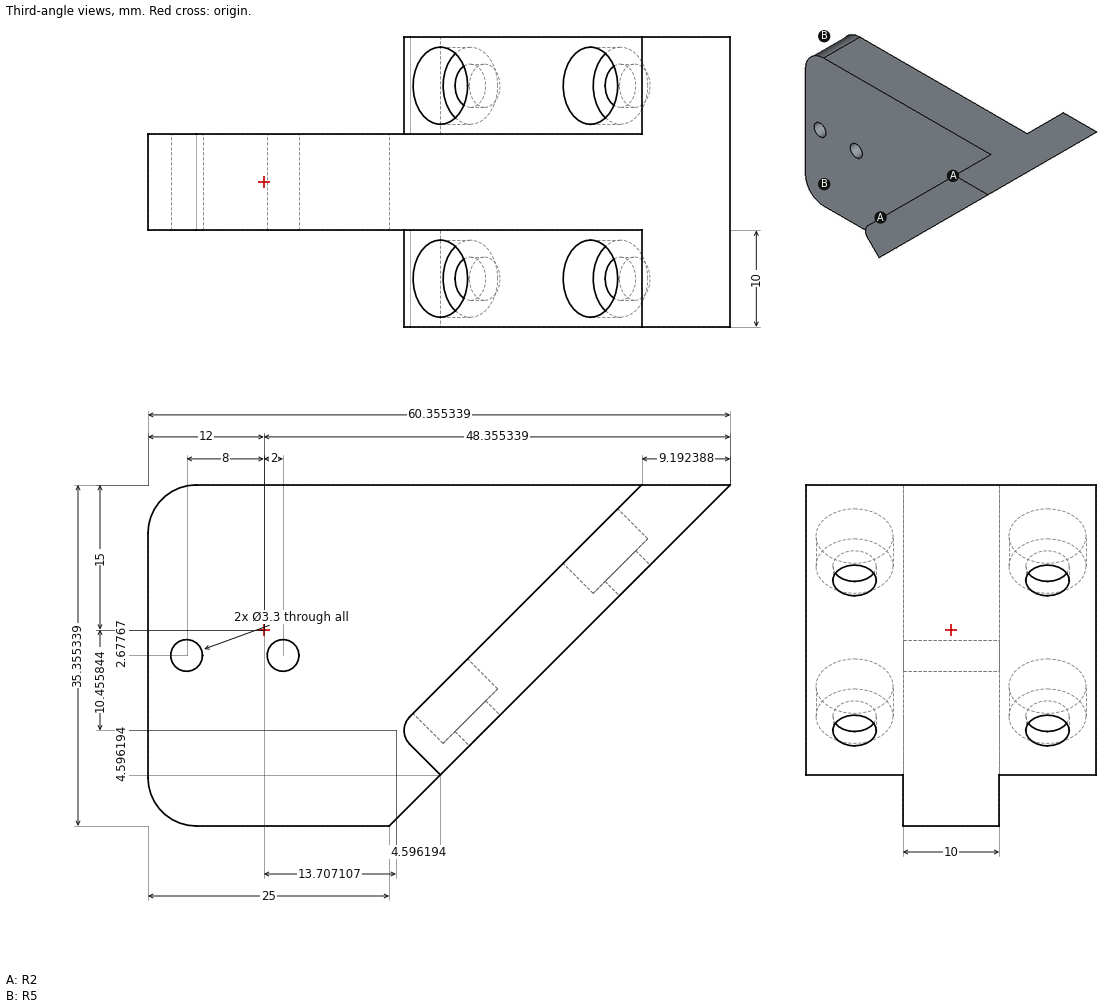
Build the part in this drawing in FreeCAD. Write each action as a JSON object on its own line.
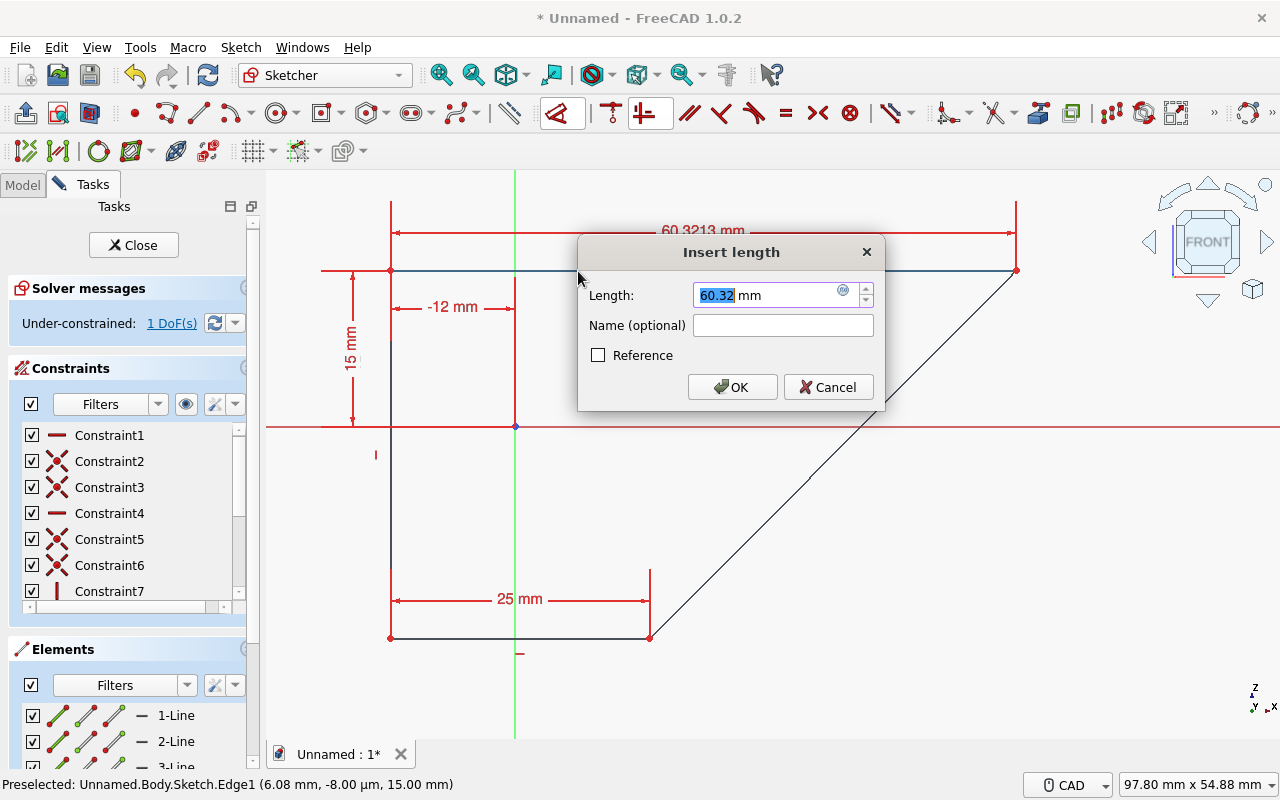
{"action": "type", "text": "60.355339"}
{"action": "key", "text": "Return"}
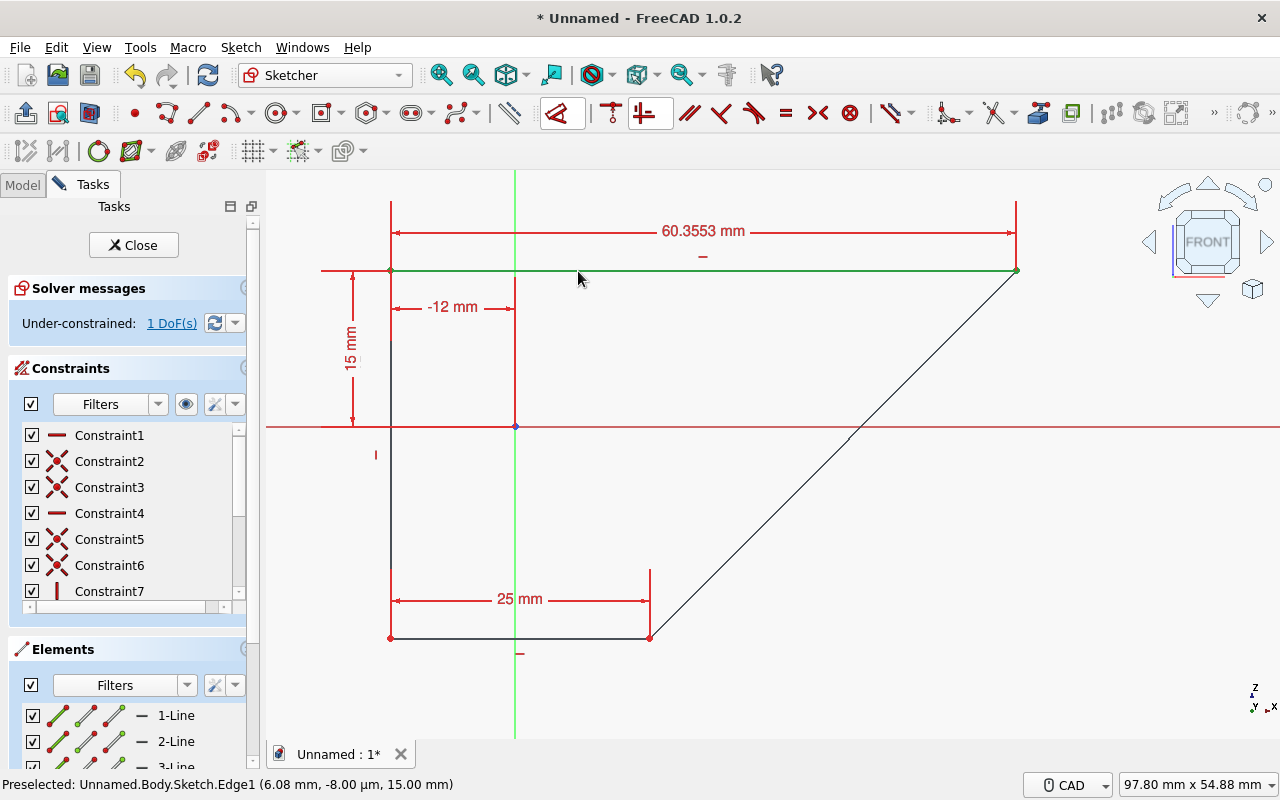
{"action": "left_click", "coordinate": [391, 529]}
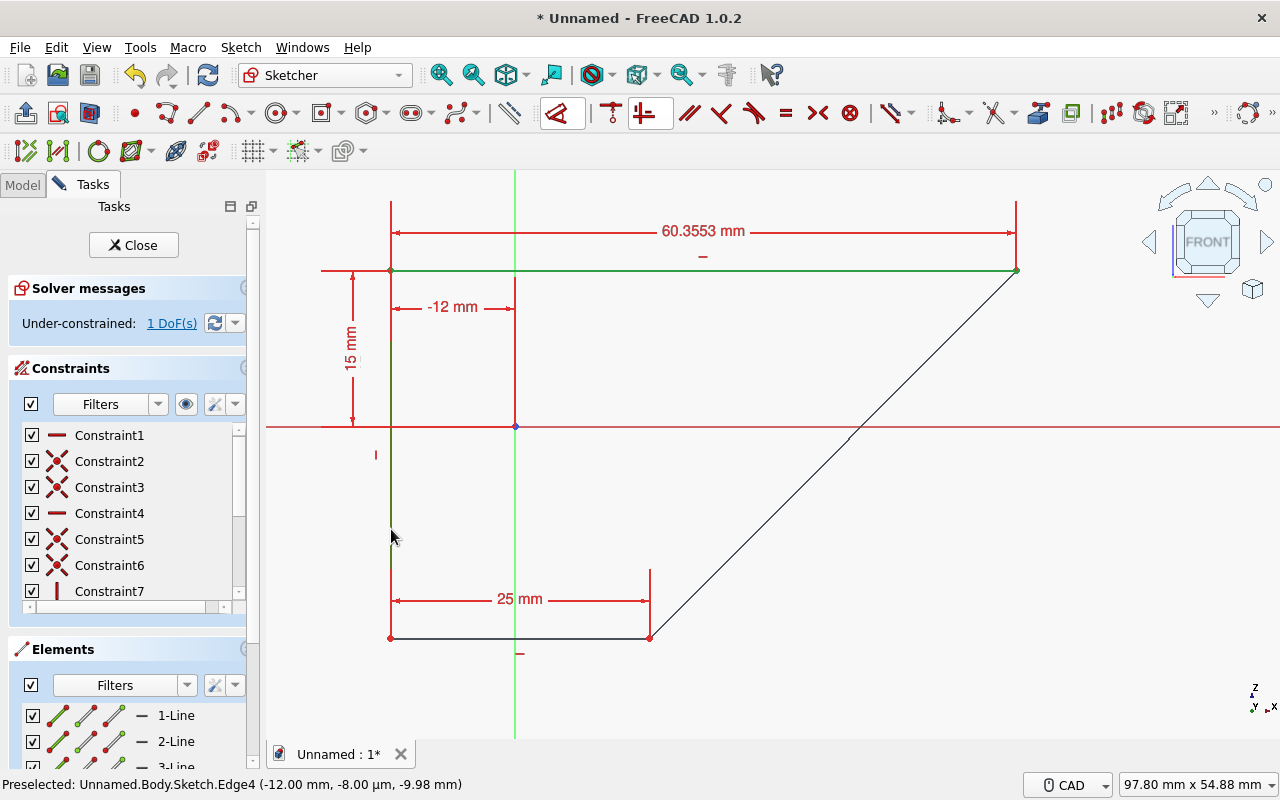
{"action": "left_click", "coordinate": [580, 114]}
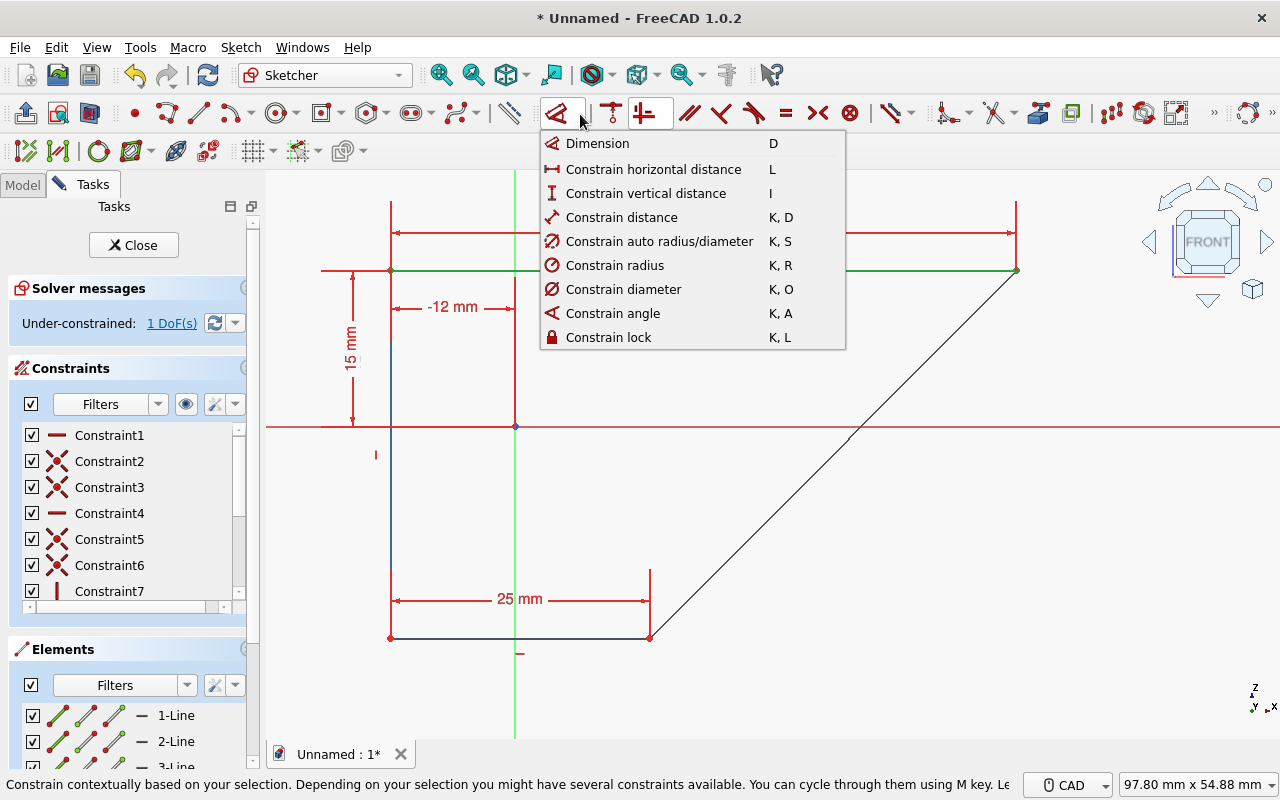
{"action": "left_click", "coordinate": [693, 193]}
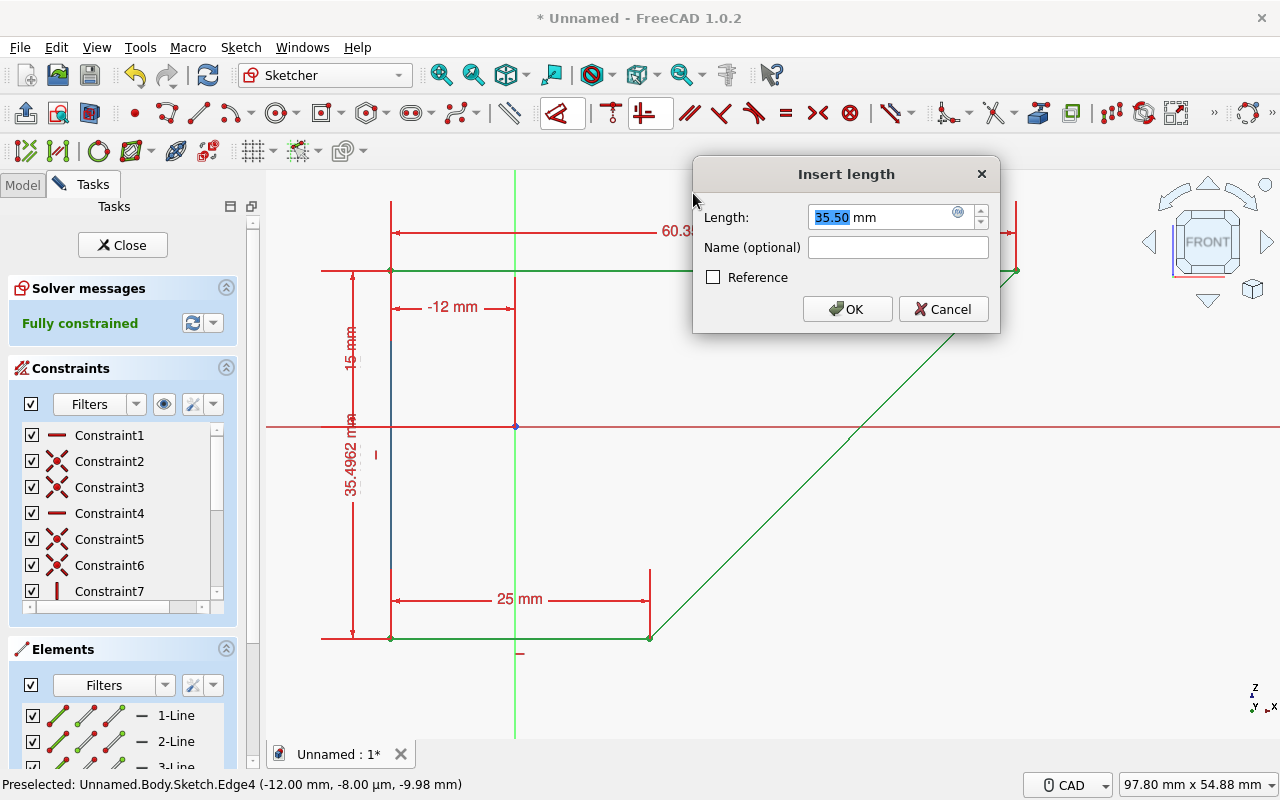
{"action": "type", "text": "35.355339"}
{"action": "key", "text": "Return"}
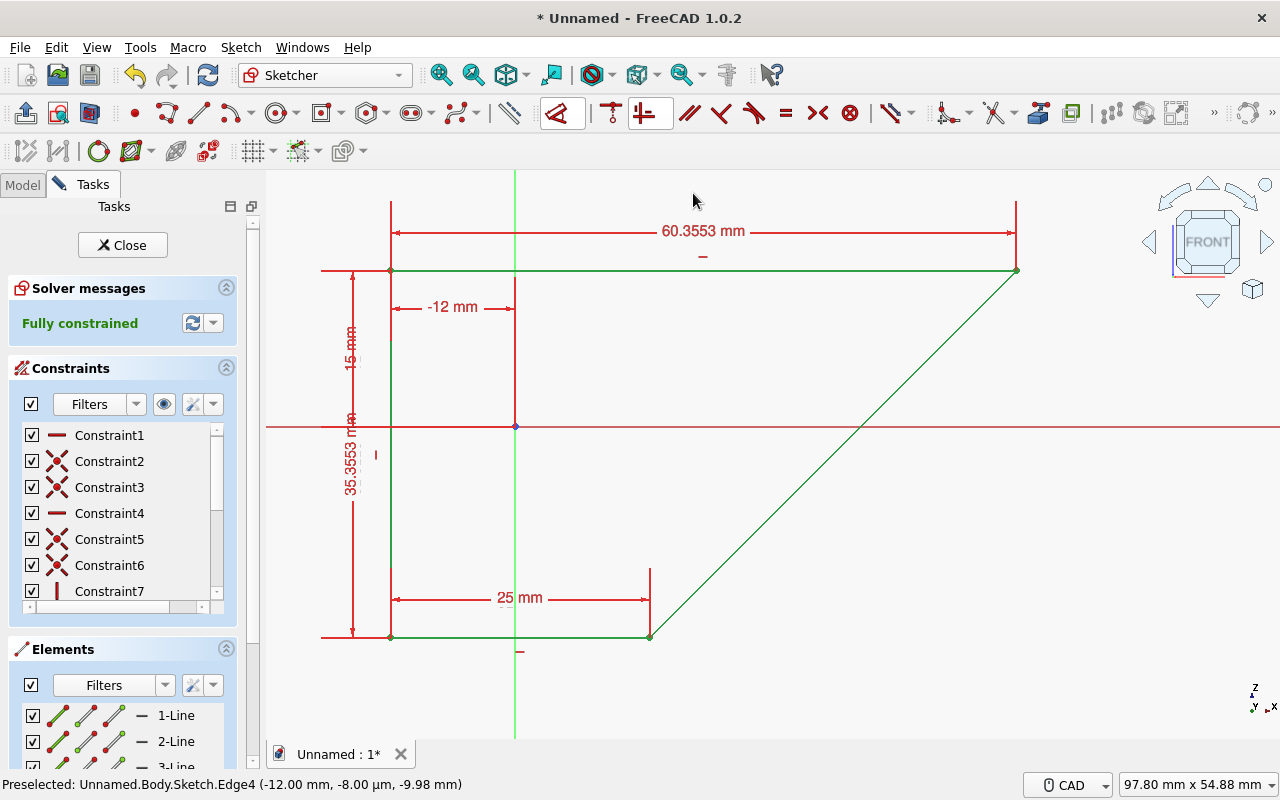
{"action": "left_click", "coordinate": [123, 245]}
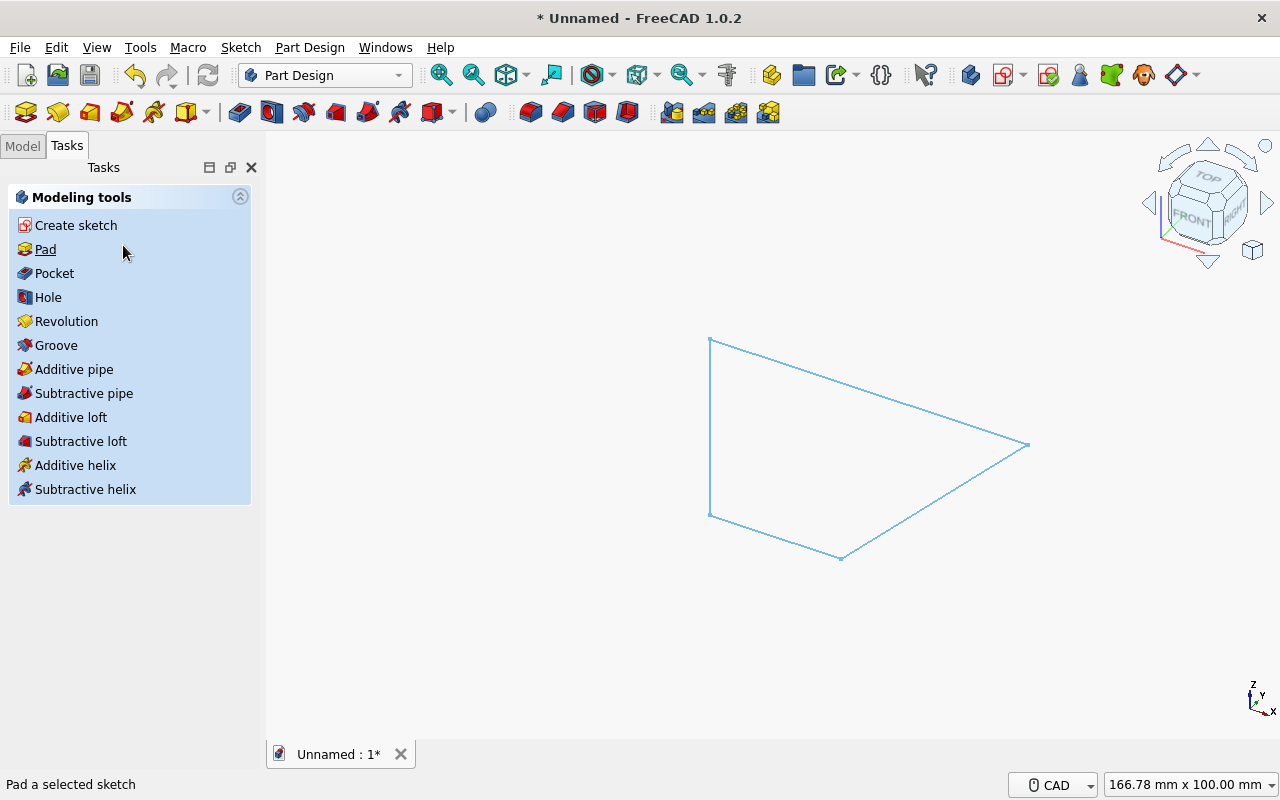
{"action": "left_click", "coordinate": [26, 112]}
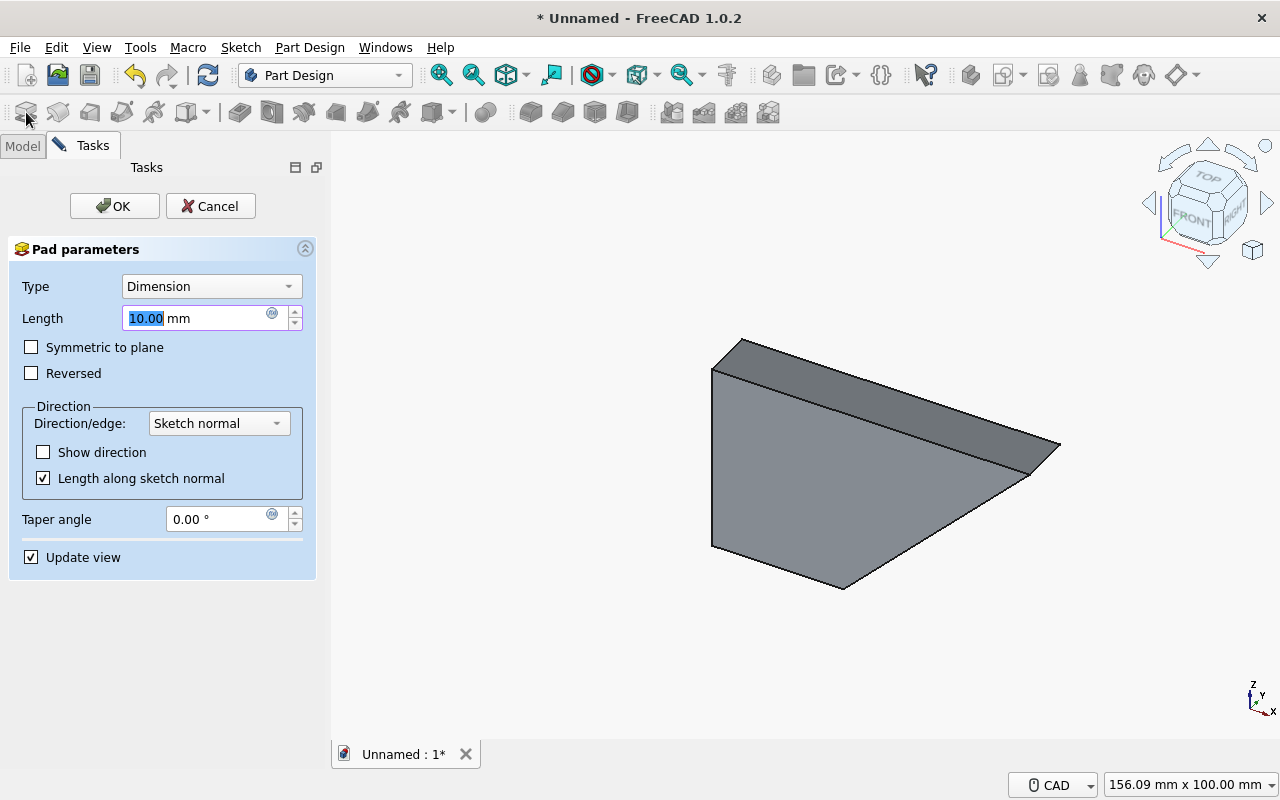
{"action": "type", "text": "10"}
{"action": "key", "text": "Tab"}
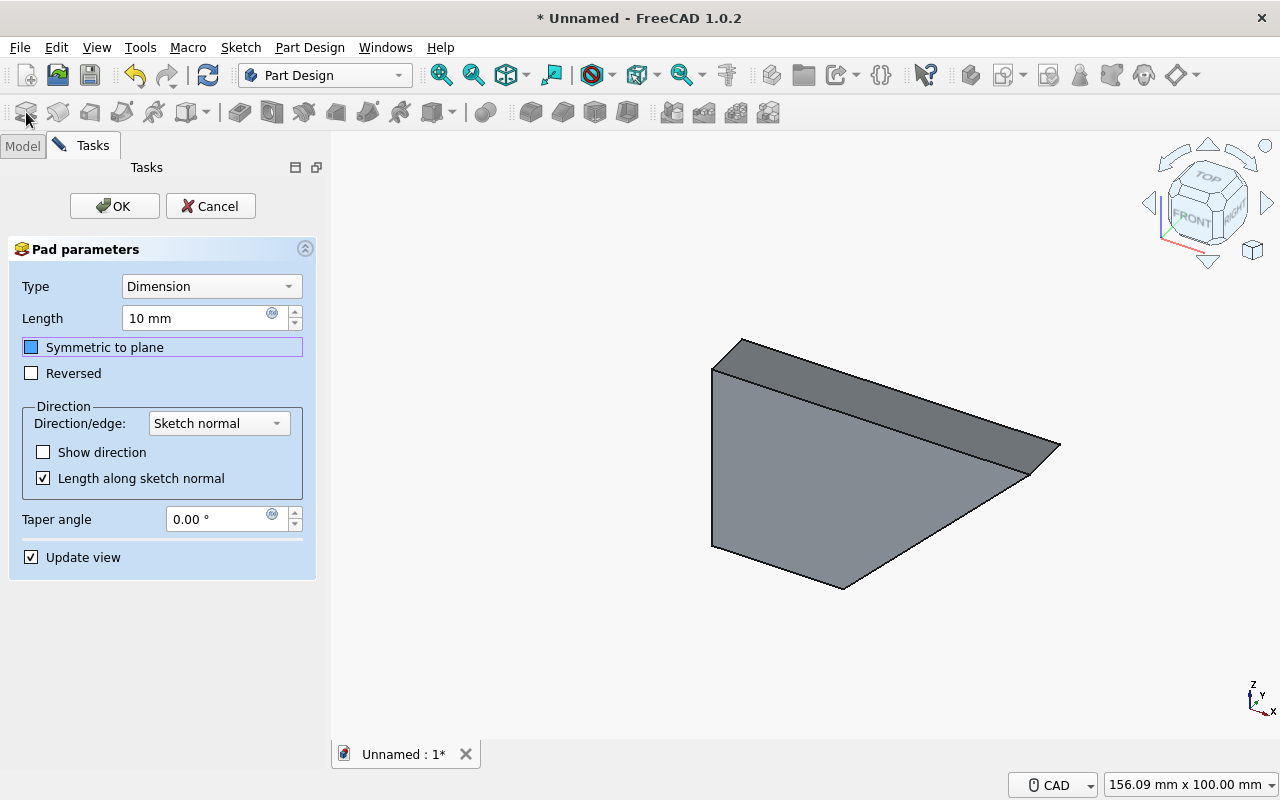
{"action": "left_click", "coordinate": [30, 347]}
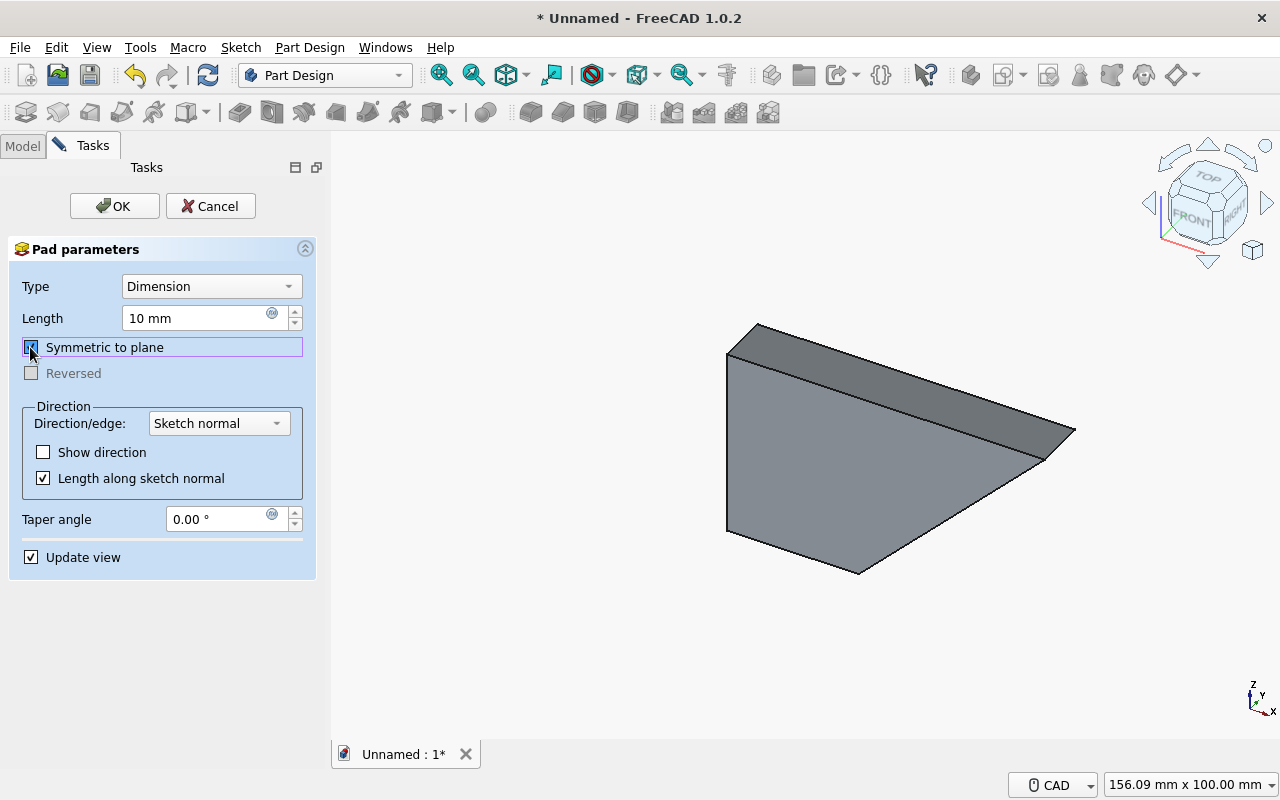
{"action": "left_click", "coordinate": [115, 206]}